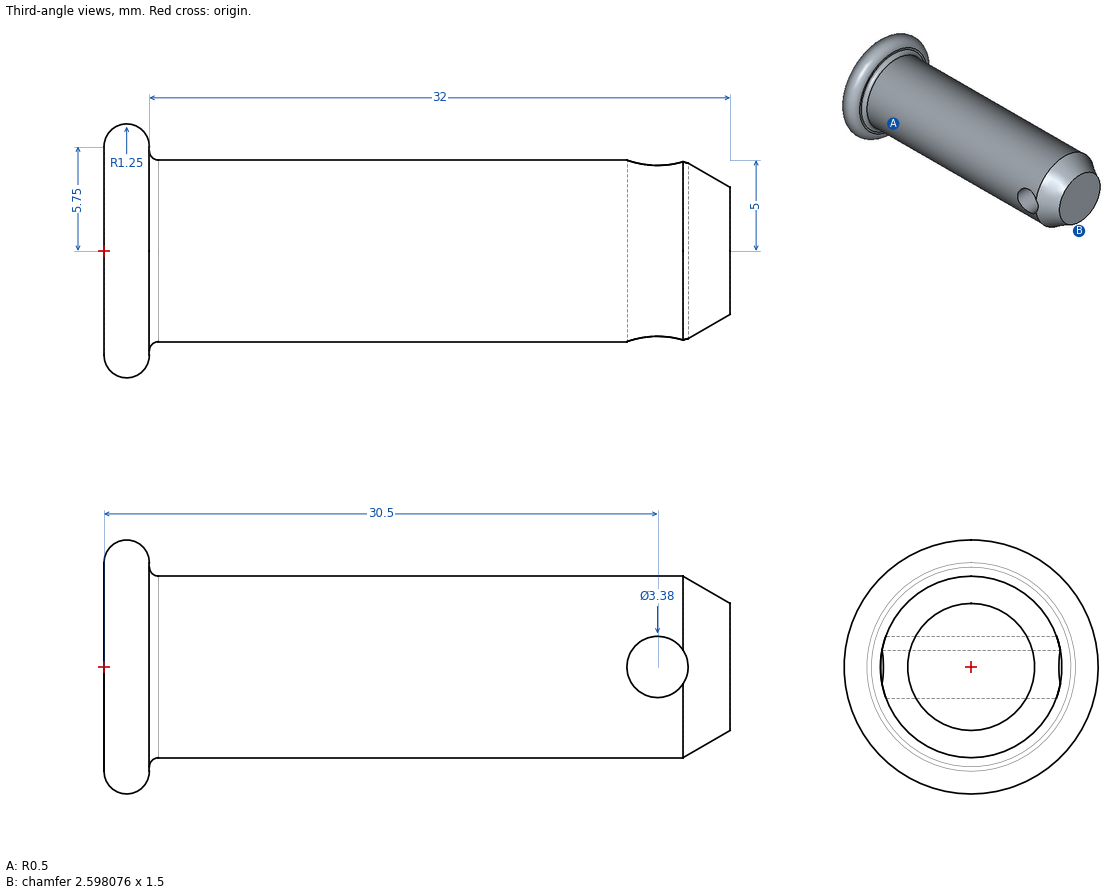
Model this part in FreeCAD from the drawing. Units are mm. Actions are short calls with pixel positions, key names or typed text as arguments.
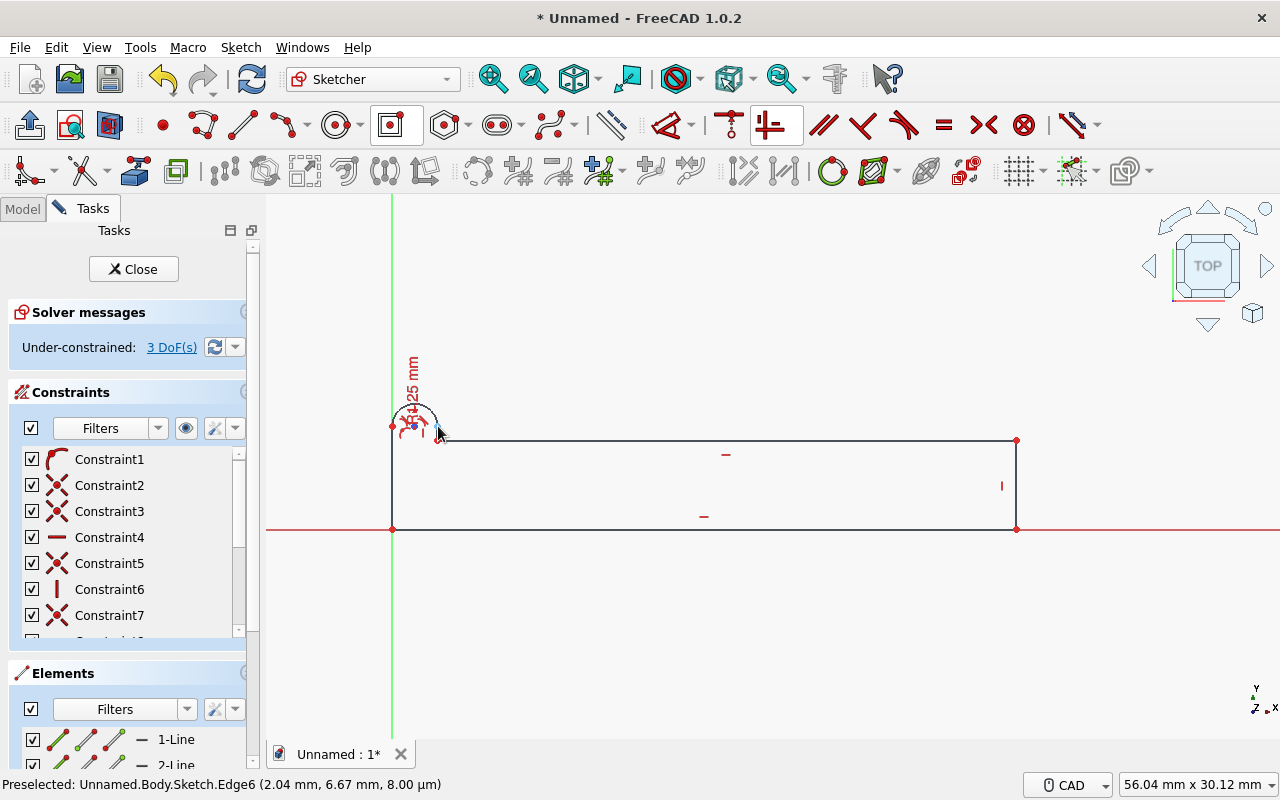
click(1016, 503)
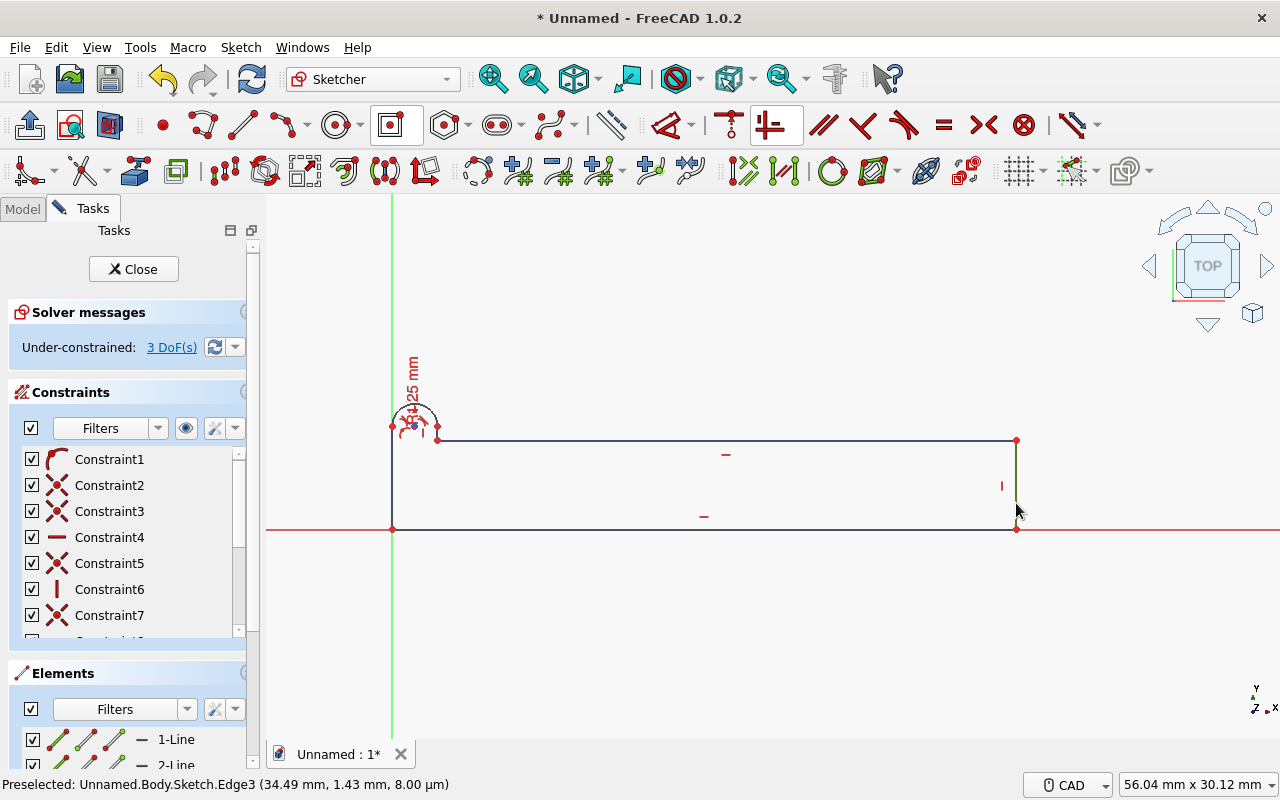
key(i)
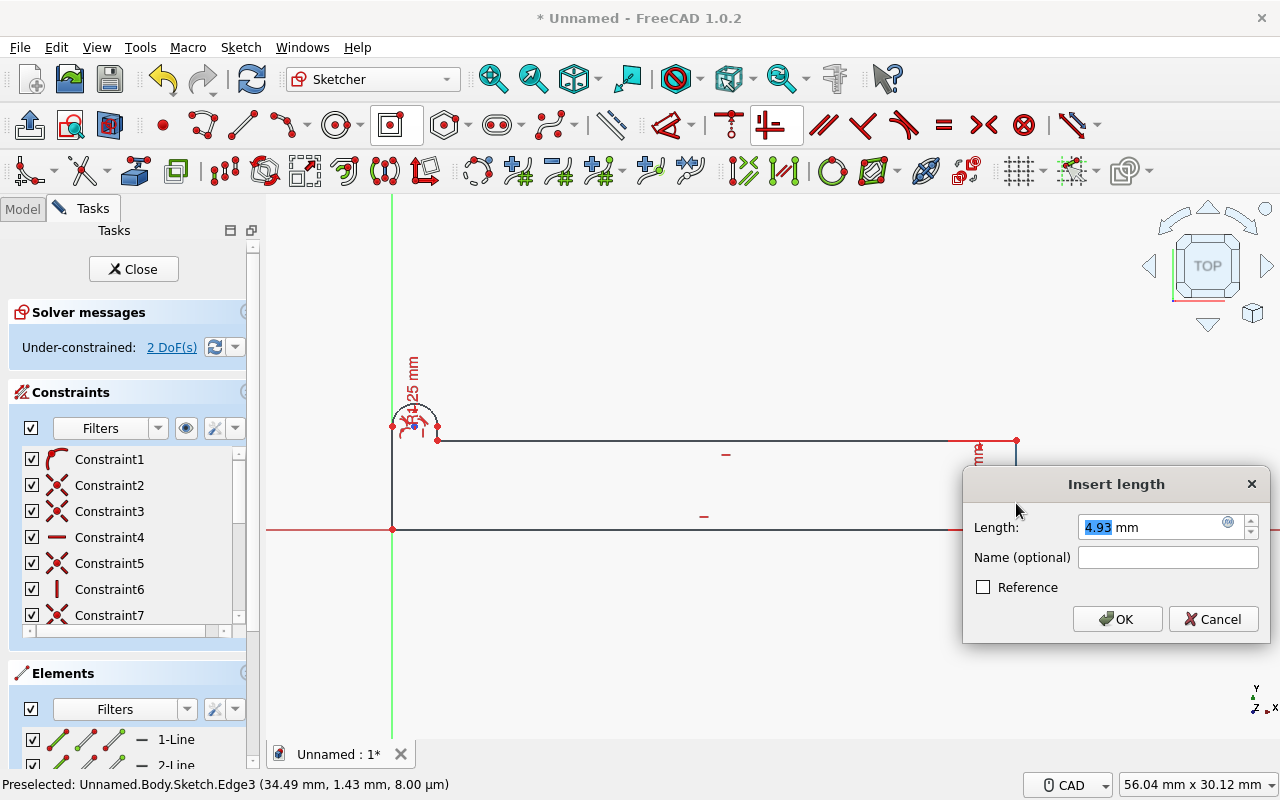
text(5)
key(Return)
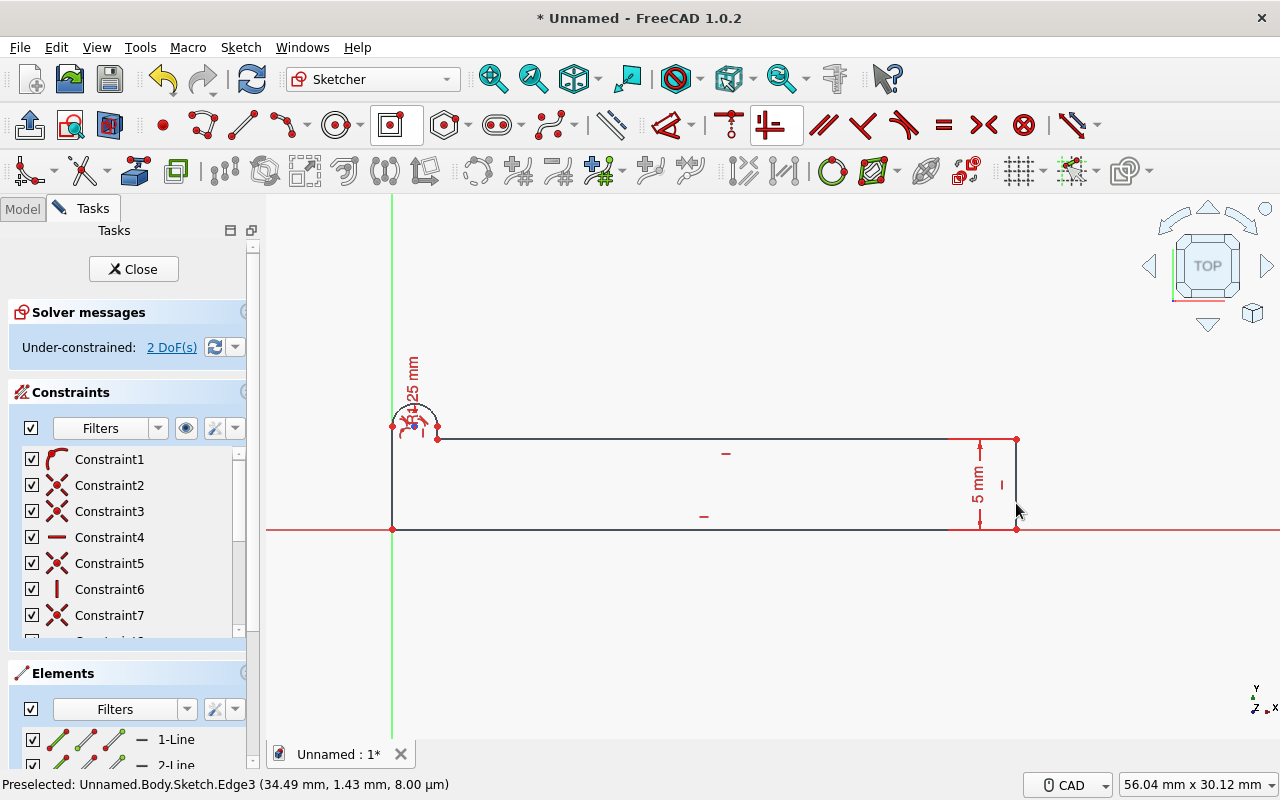
click(843, 439)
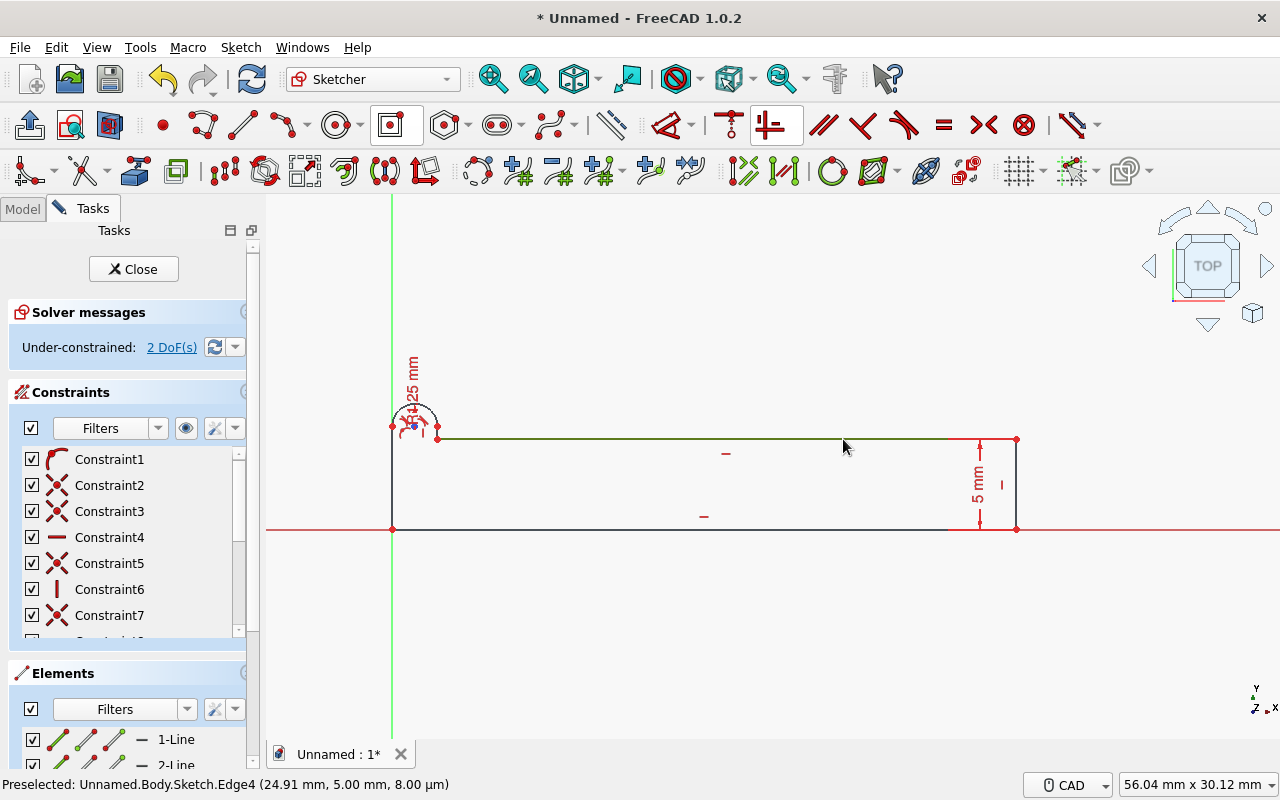
key(l)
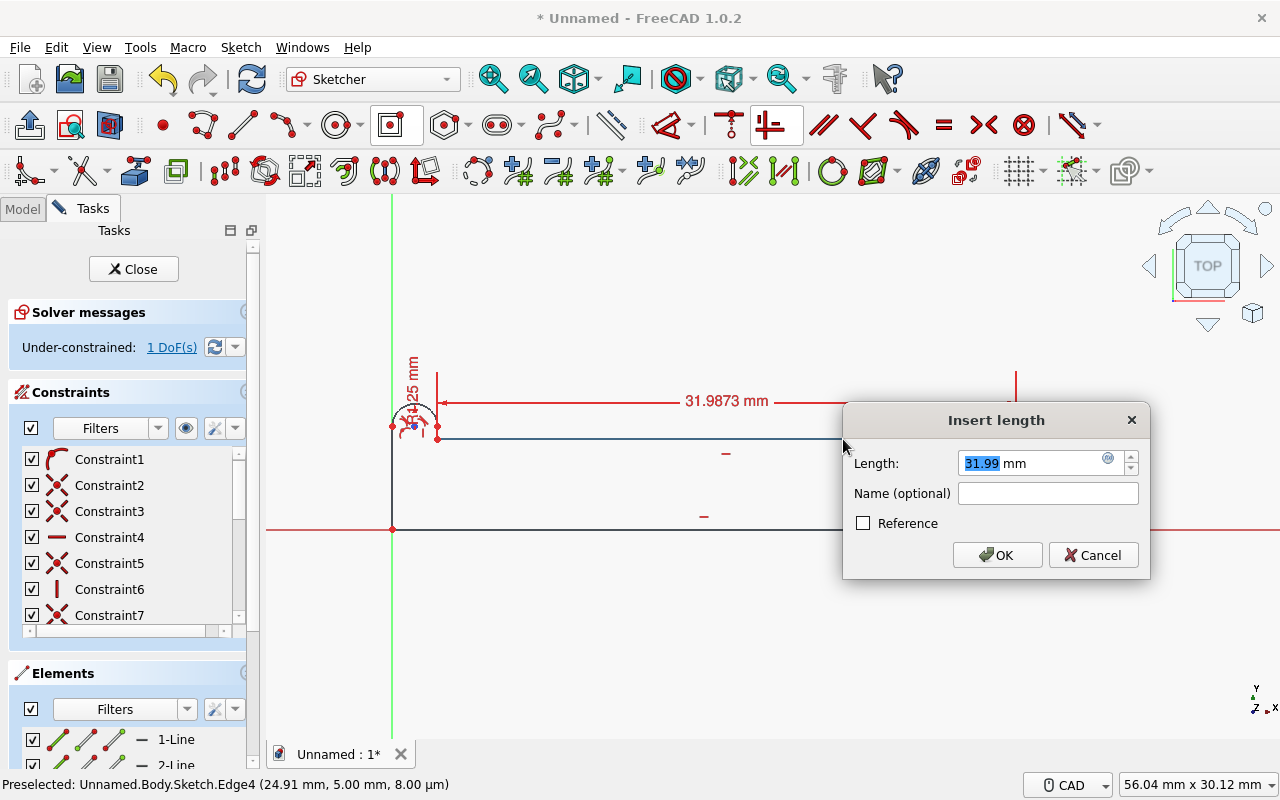
text(32)
key(Return)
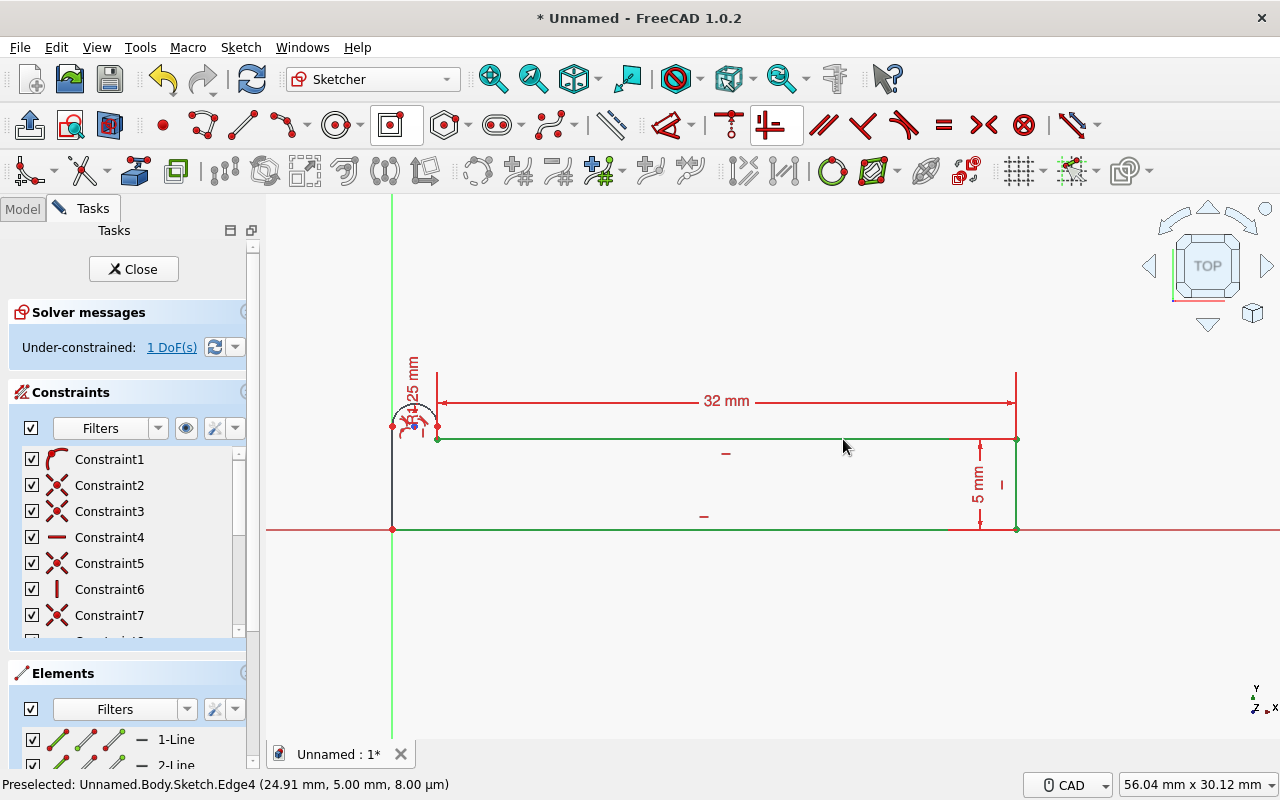
click(392, 458)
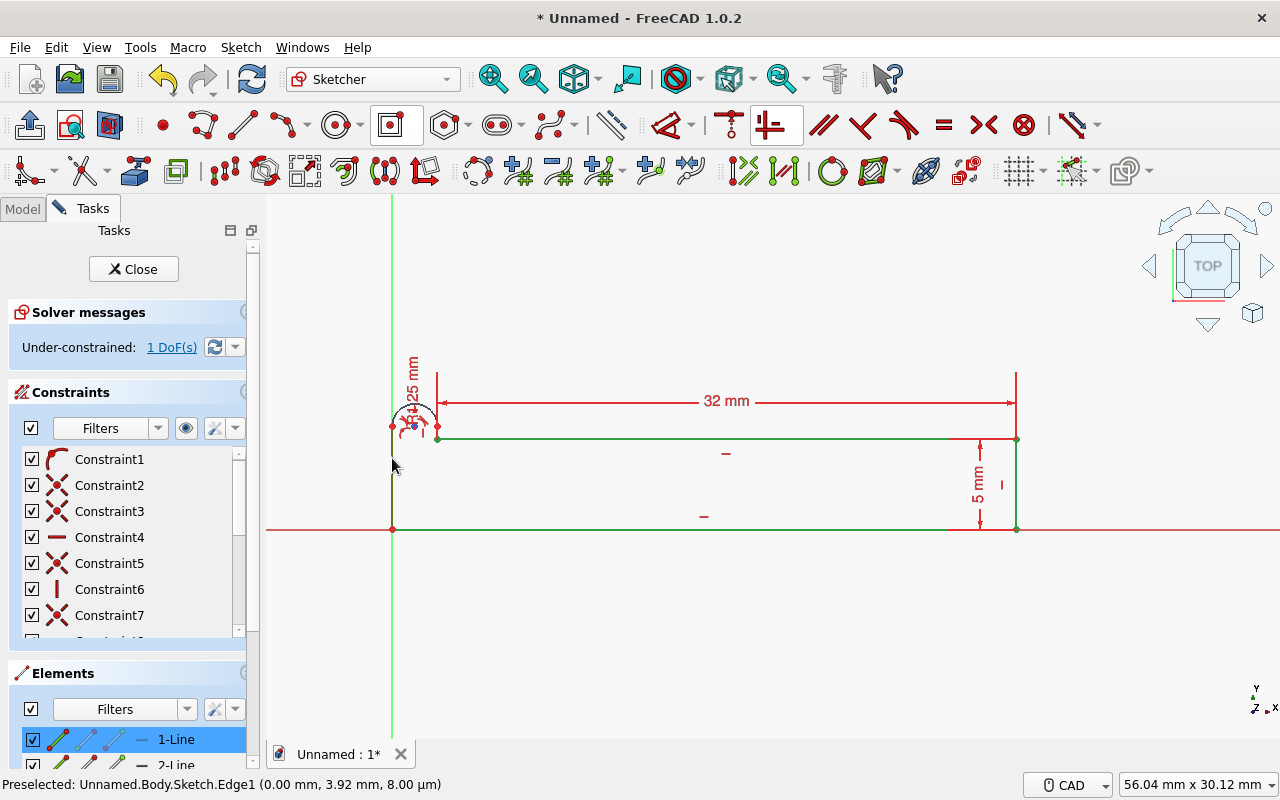
key(i)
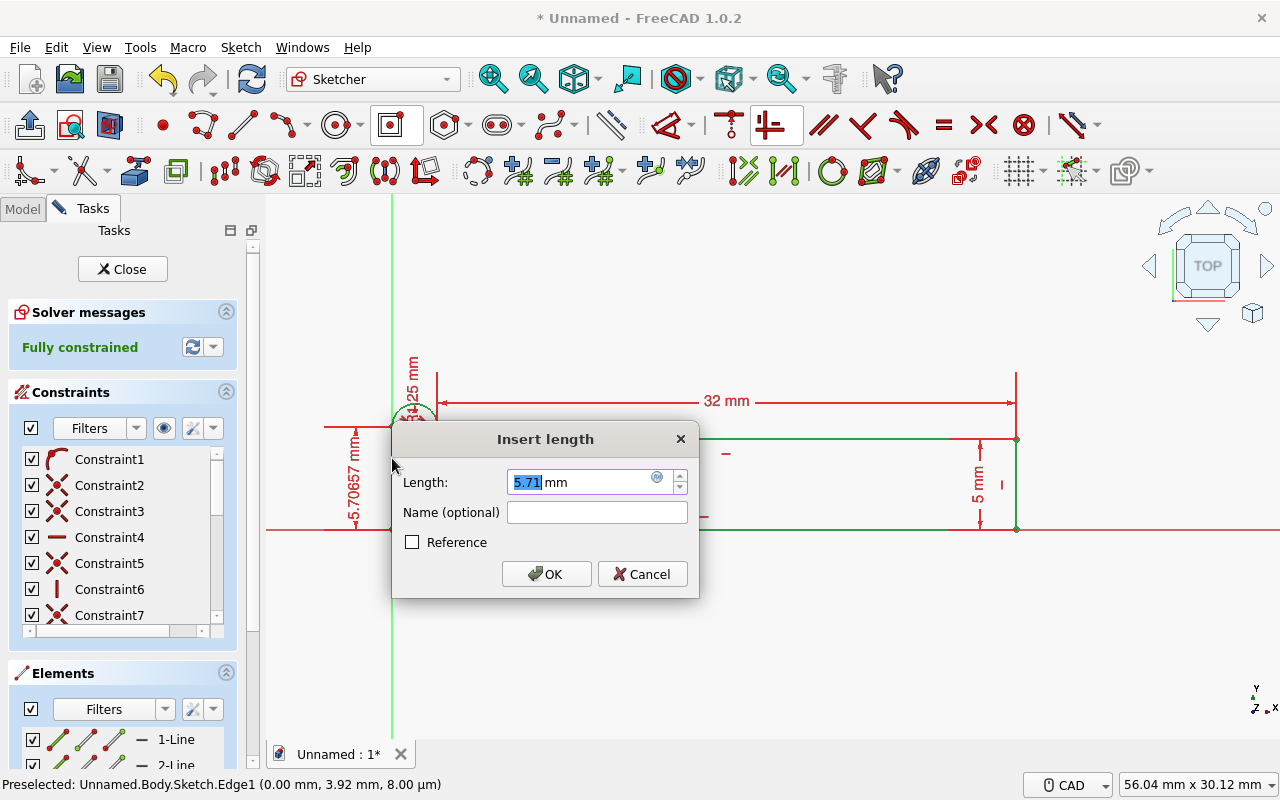
text(5.75)
key(Return)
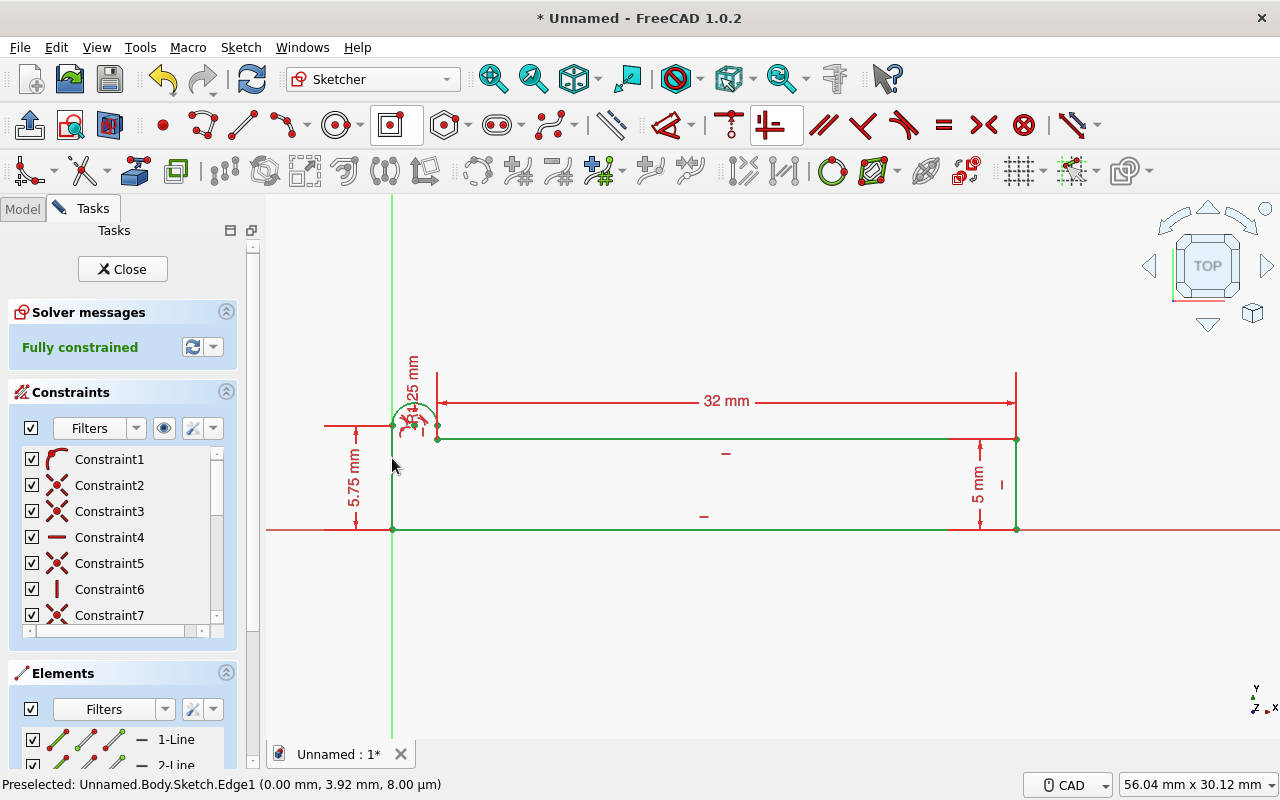
click(123, 269)